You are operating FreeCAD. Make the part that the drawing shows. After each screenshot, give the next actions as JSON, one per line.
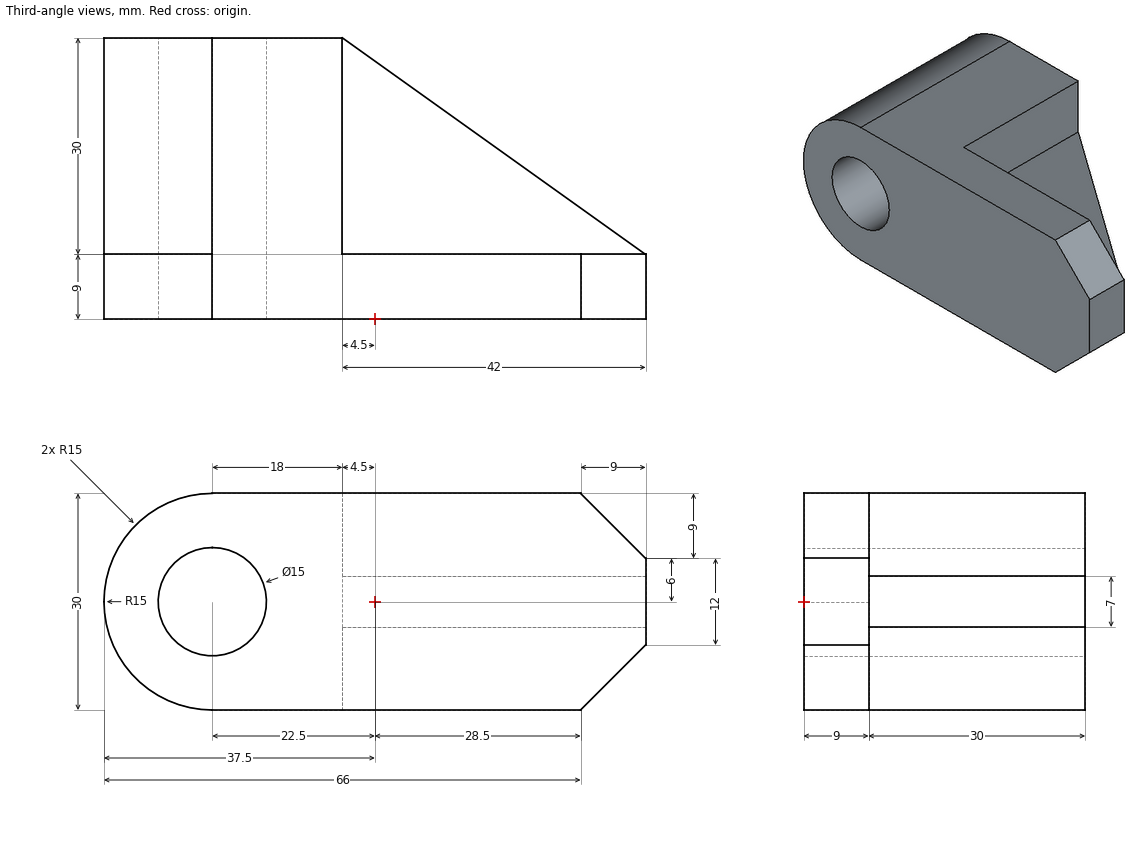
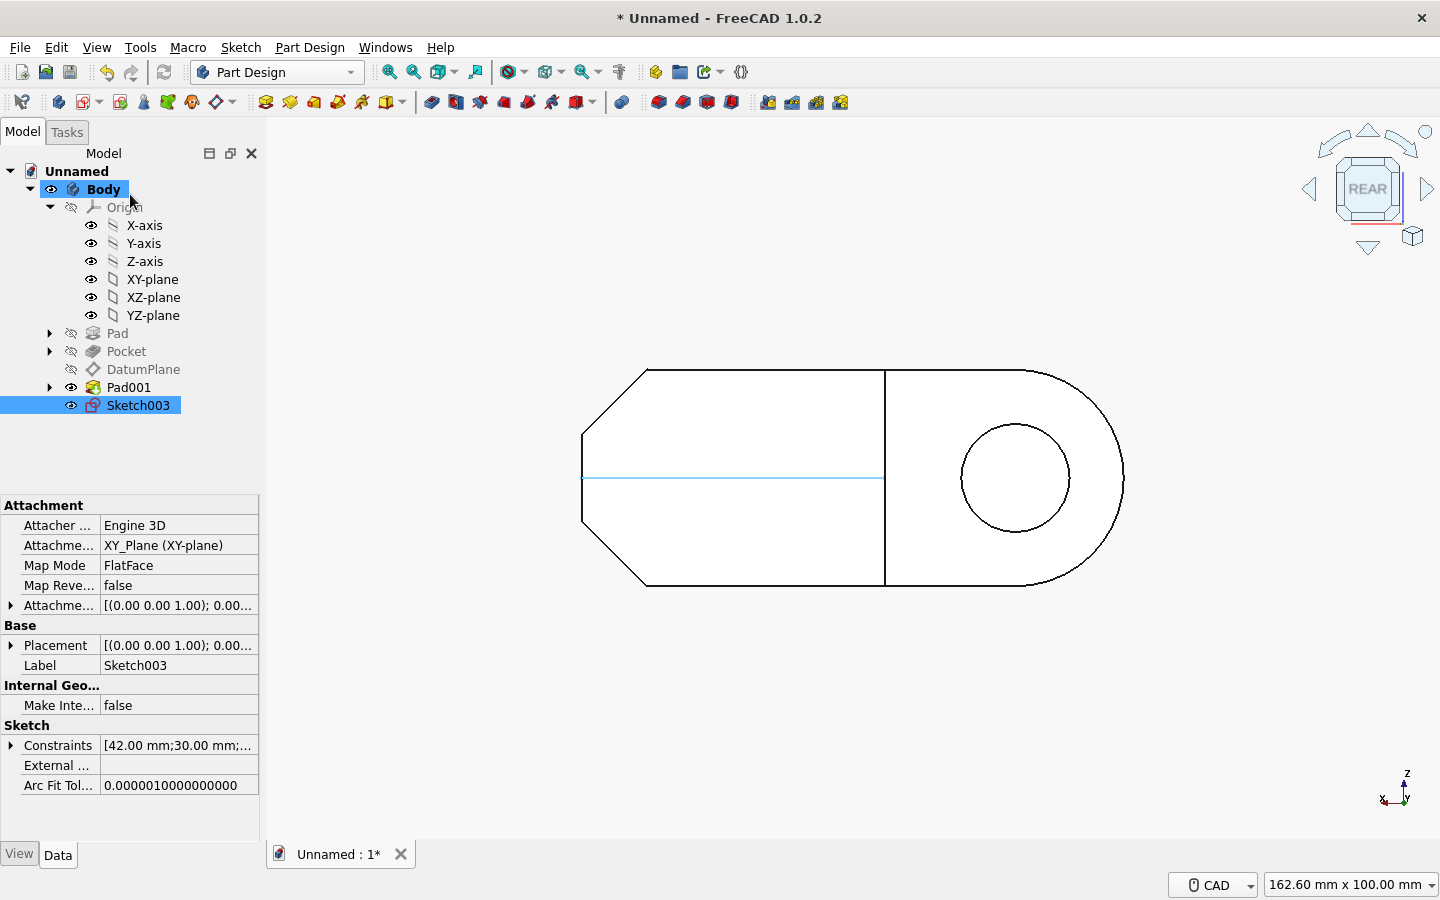
{"action": "left_click", "coordinate": [266, 102]}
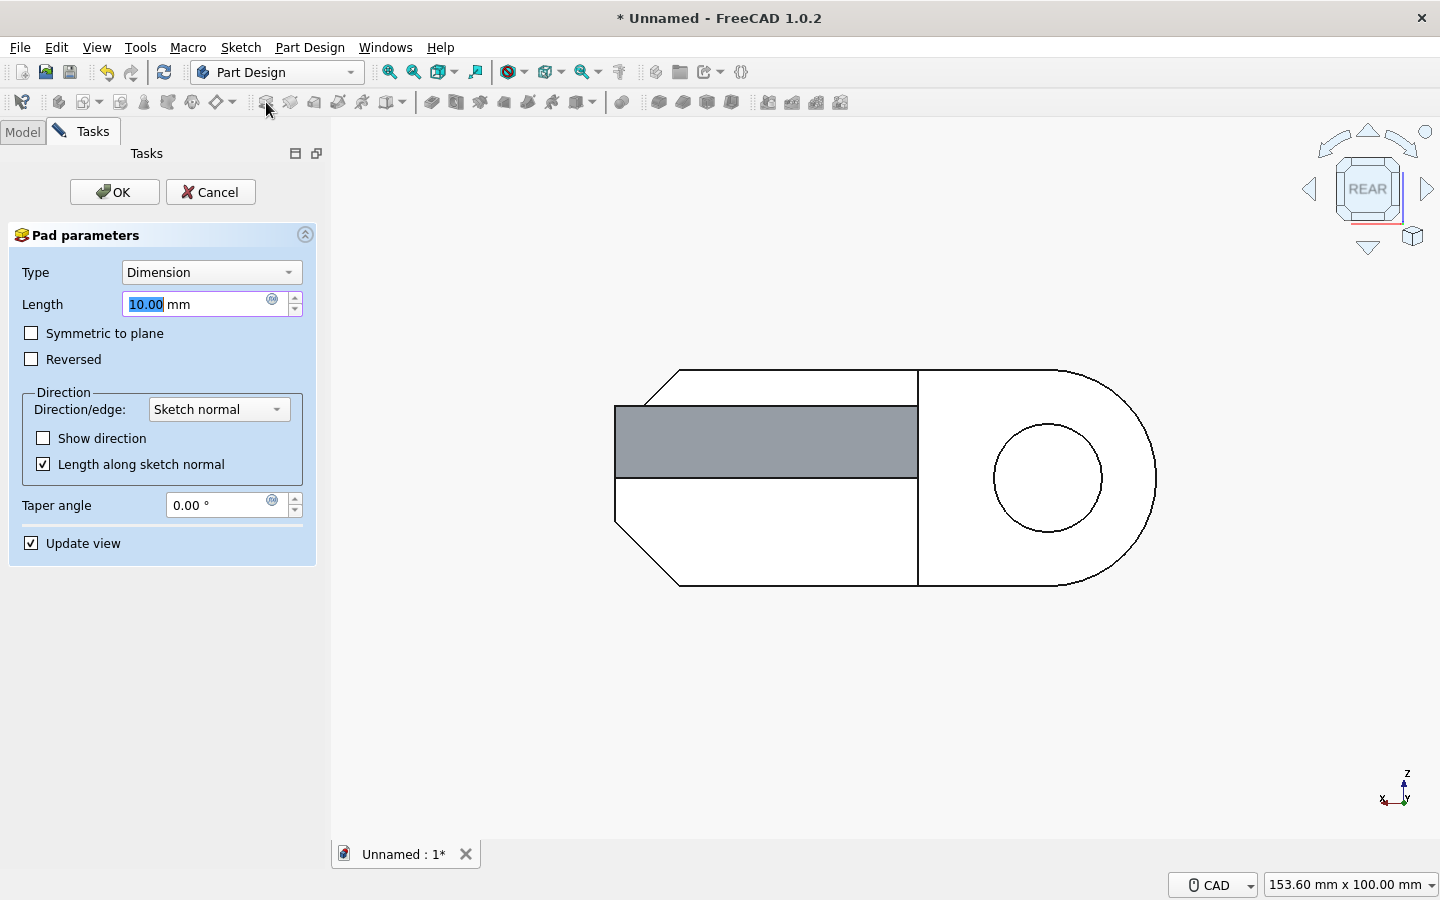
{"action": "type", "text": "7"}
{"action": "key", "text": "Tab"}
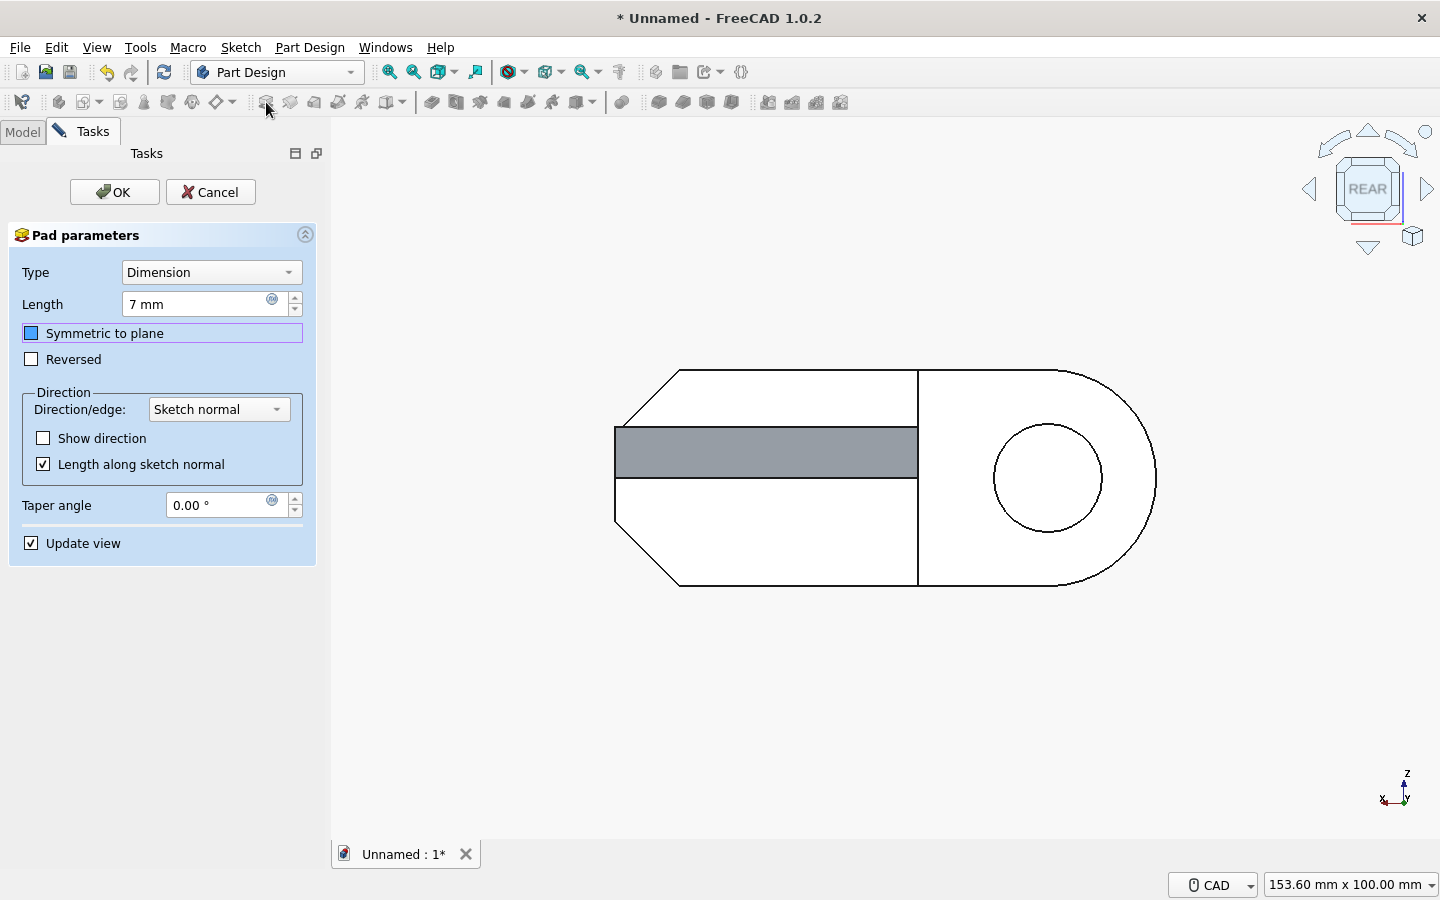
{"action": "left_click", "coordinate": [30, 333]}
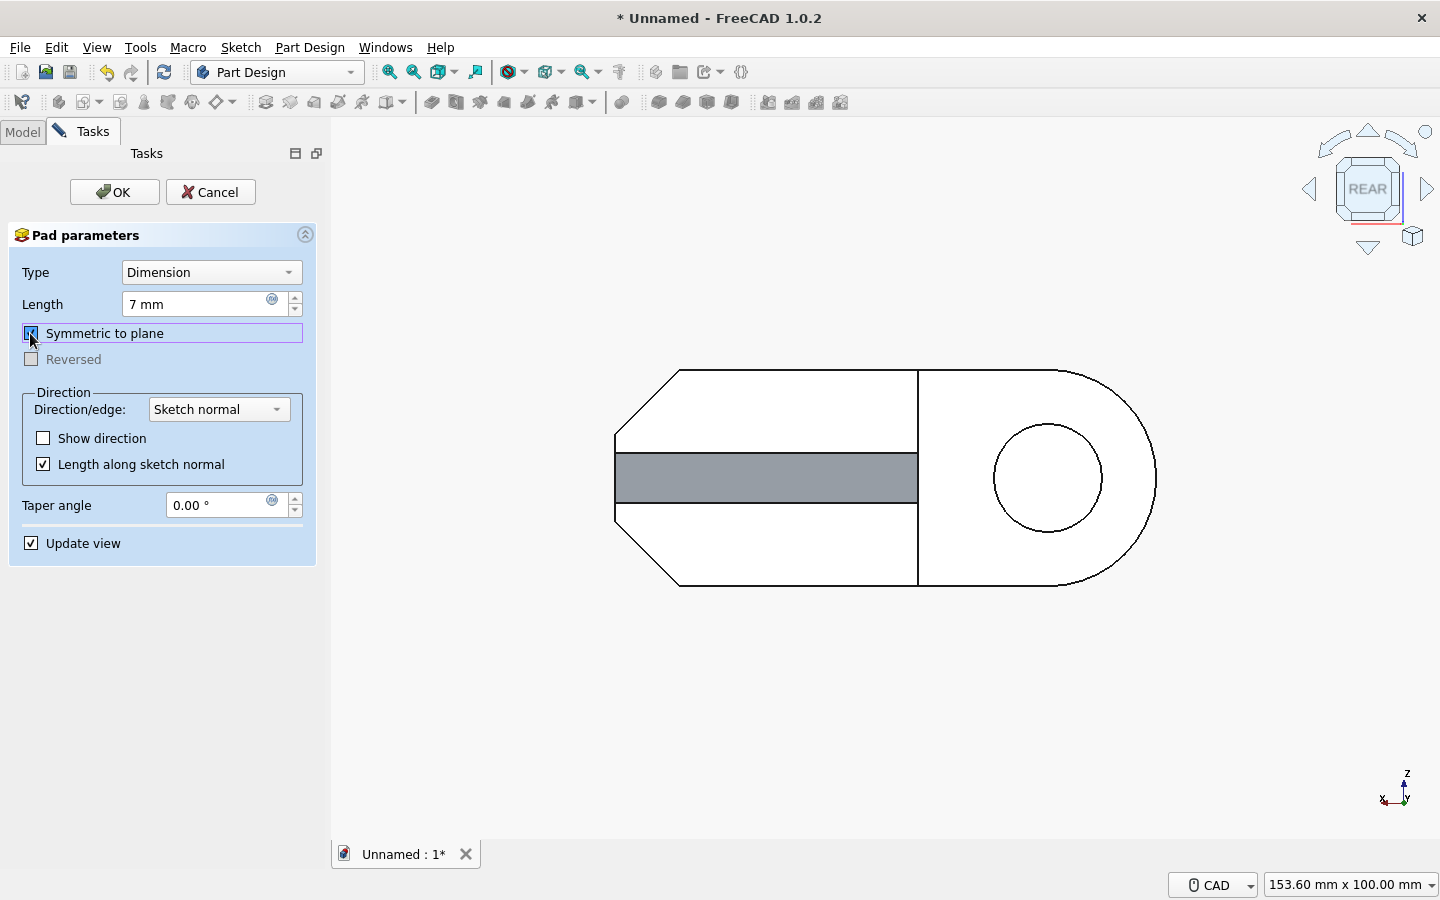
{"action": "left_click", "coordinate": [115, 192]}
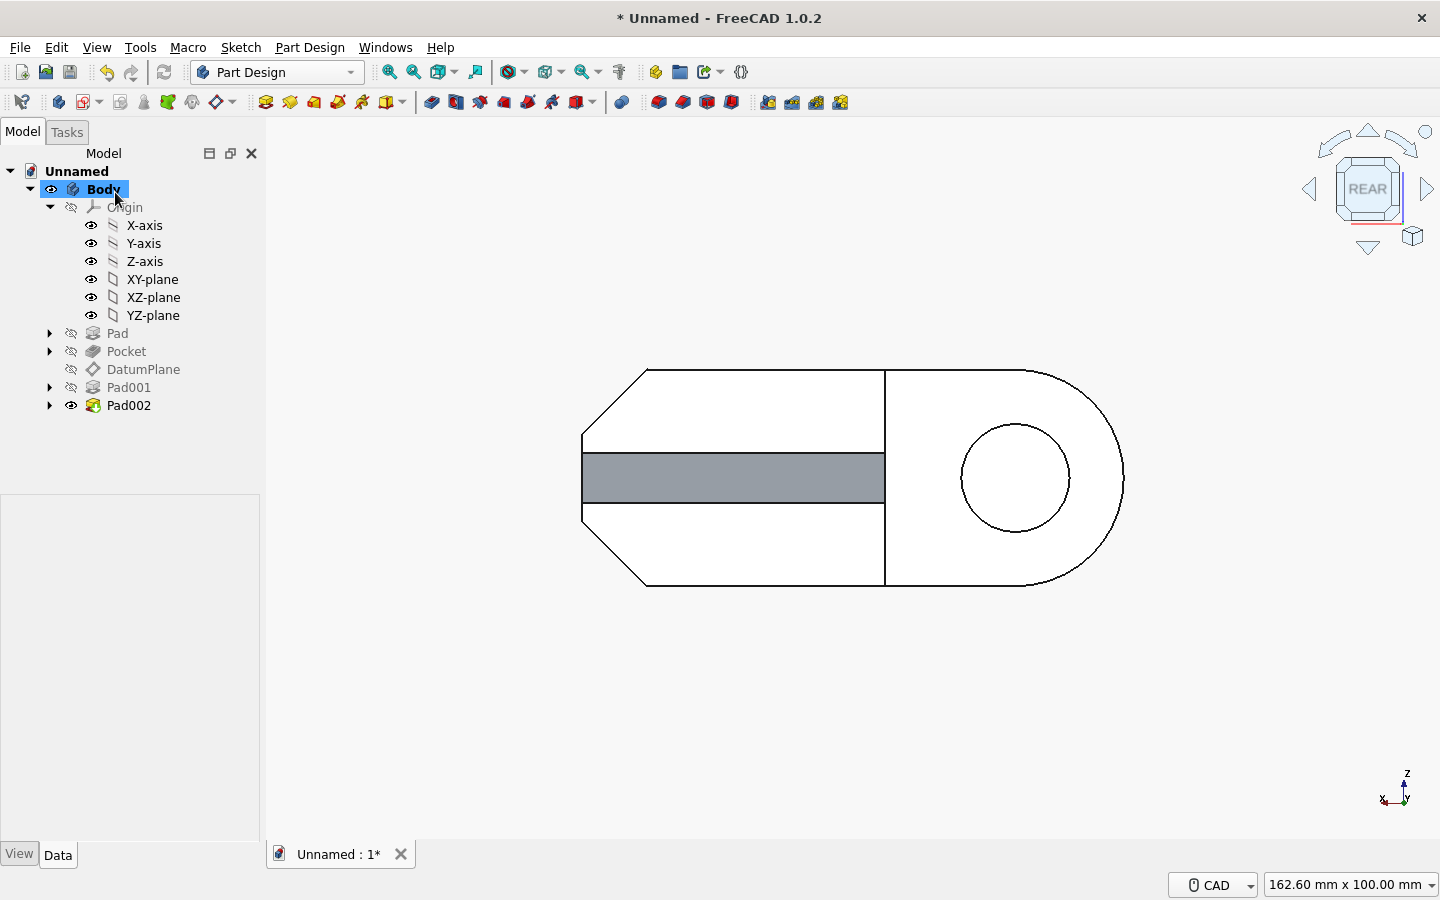
{"action": "left_click", "coordinate": [937, 415]}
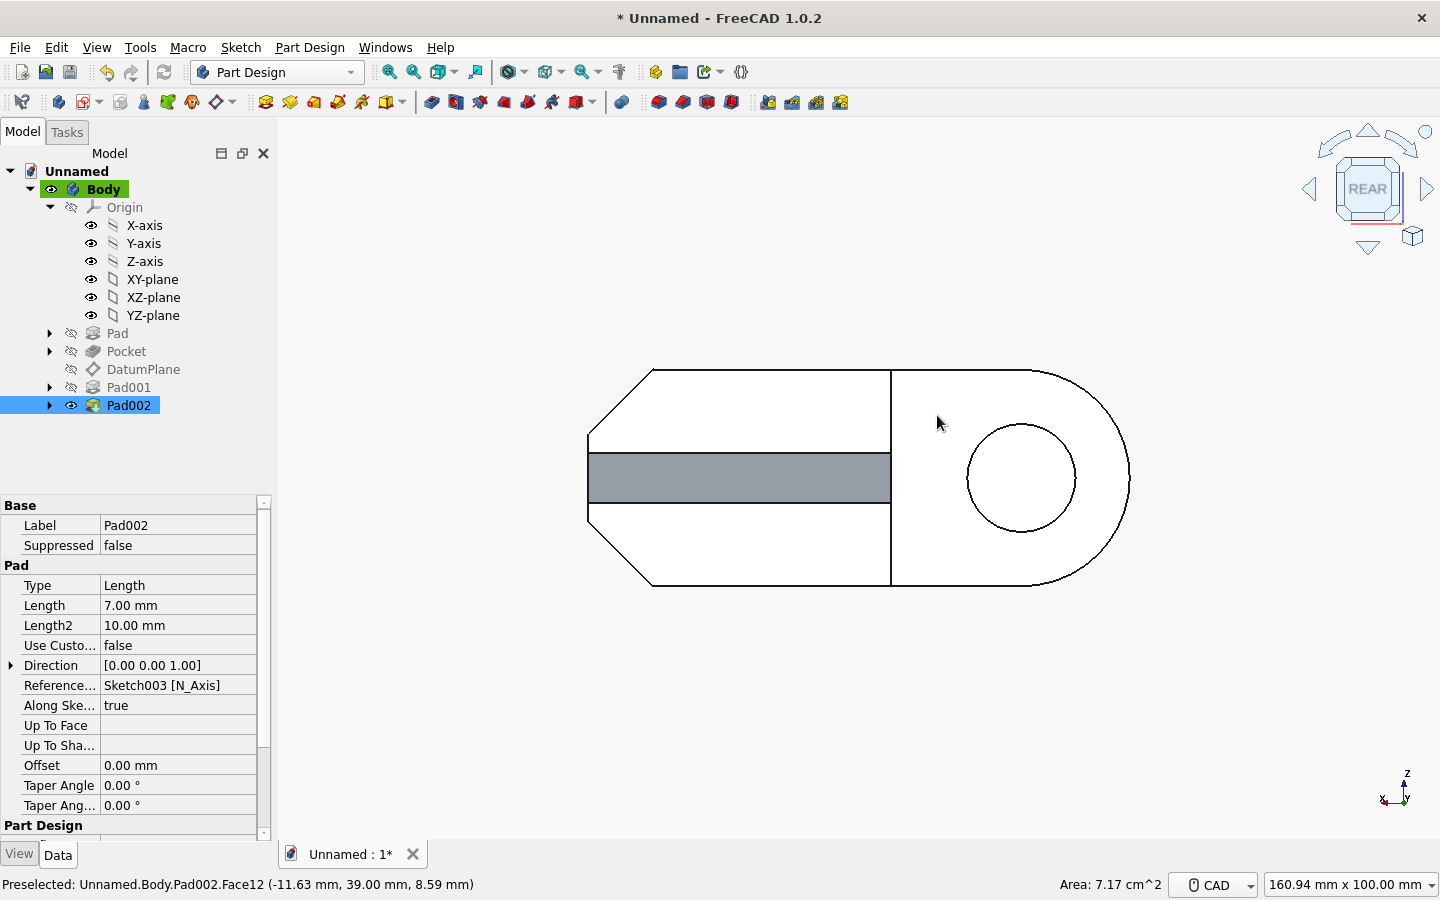
{"action": "left_click", "coordinate": [84, 102]}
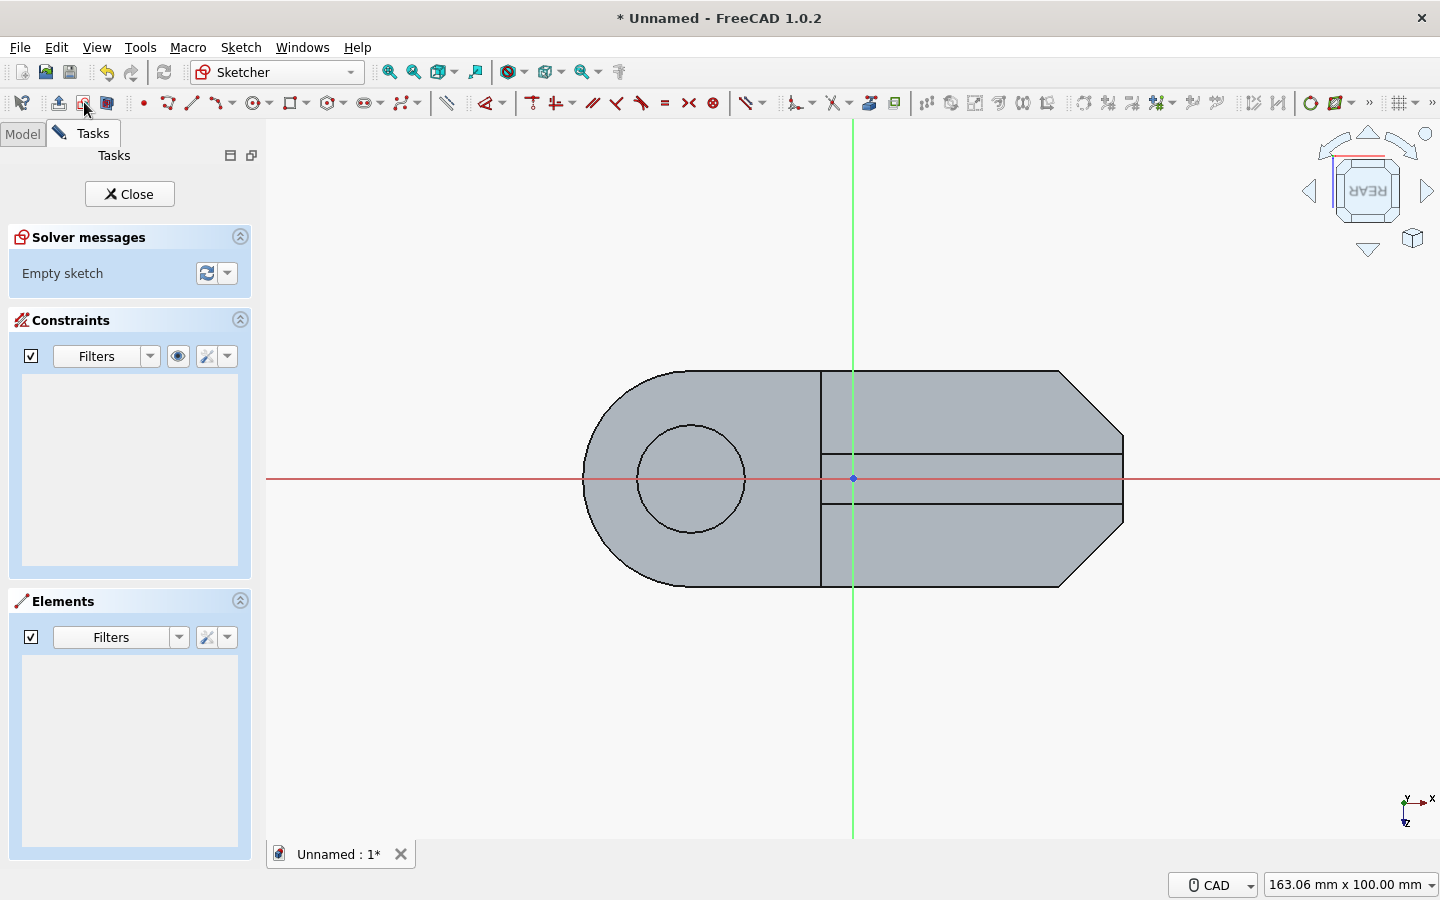
{"action": "scroll", "coordinate": [728, 479], "scroll_direction": "up", "scroll_amount": 6}